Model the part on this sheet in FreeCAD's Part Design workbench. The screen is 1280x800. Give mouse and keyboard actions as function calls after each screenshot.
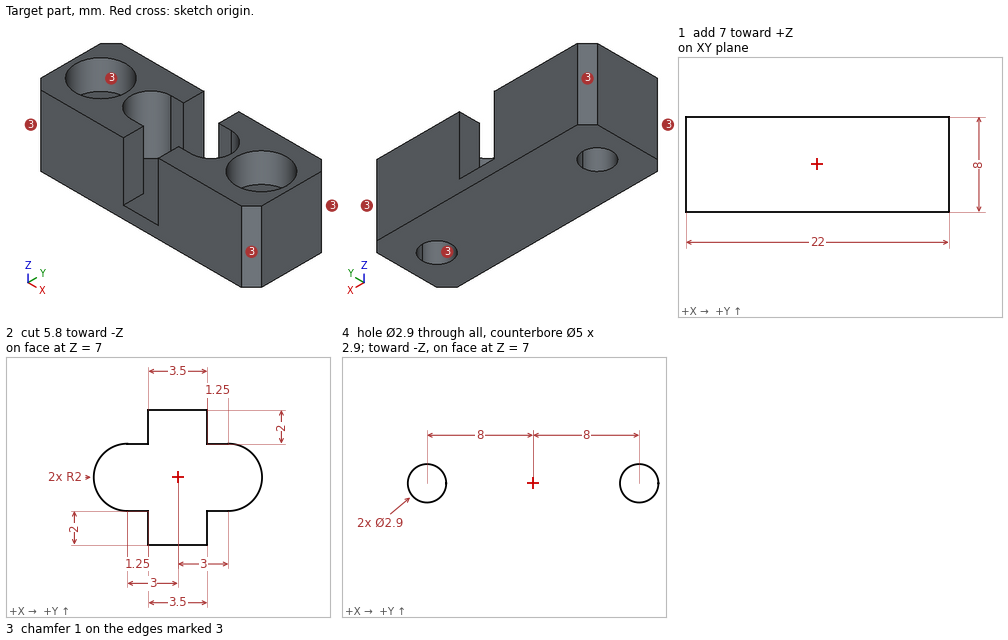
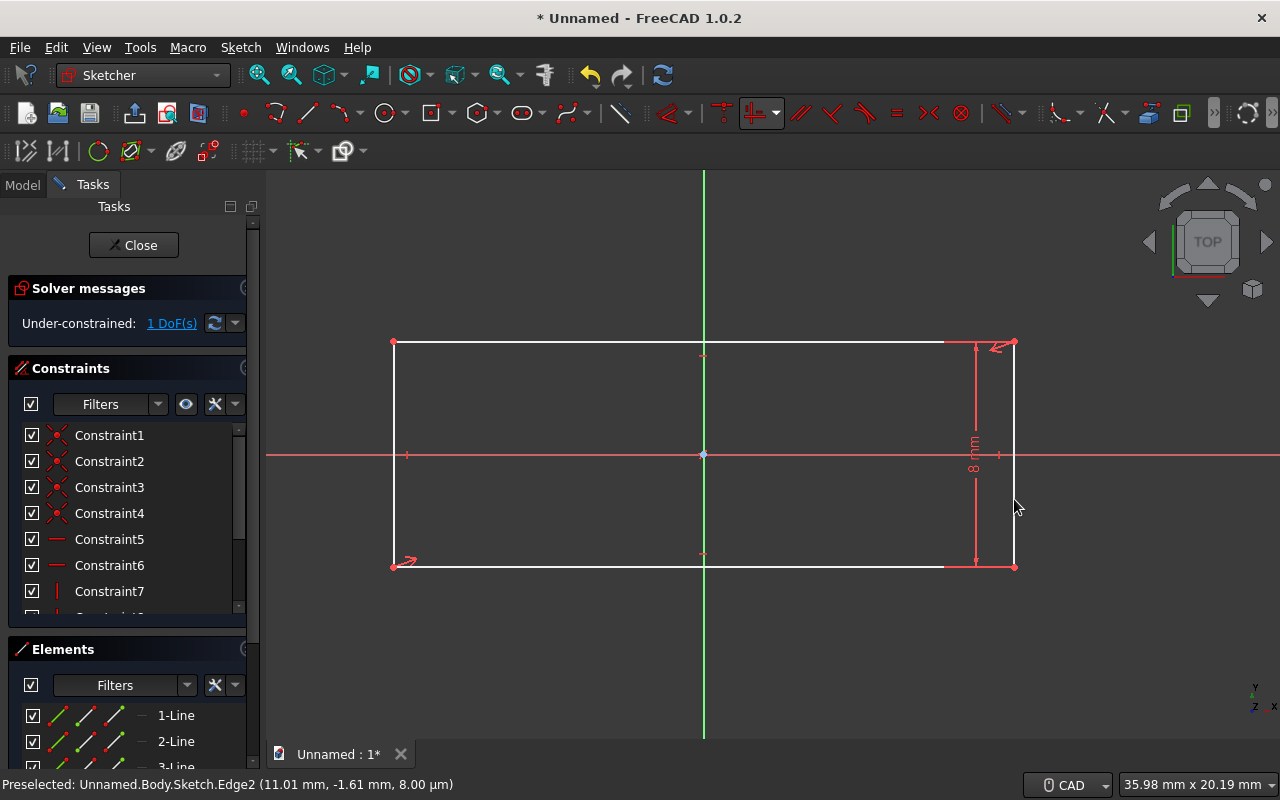
click(580, 567)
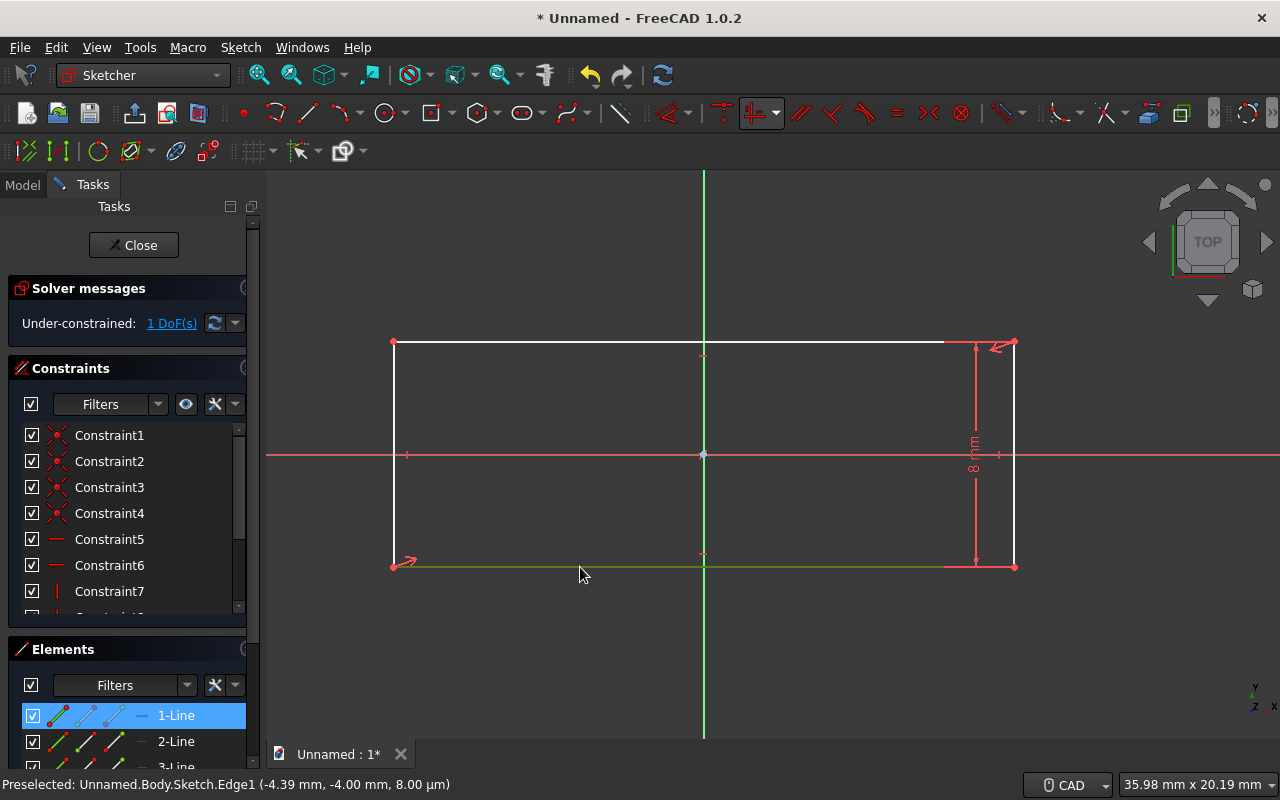
click(690, 114)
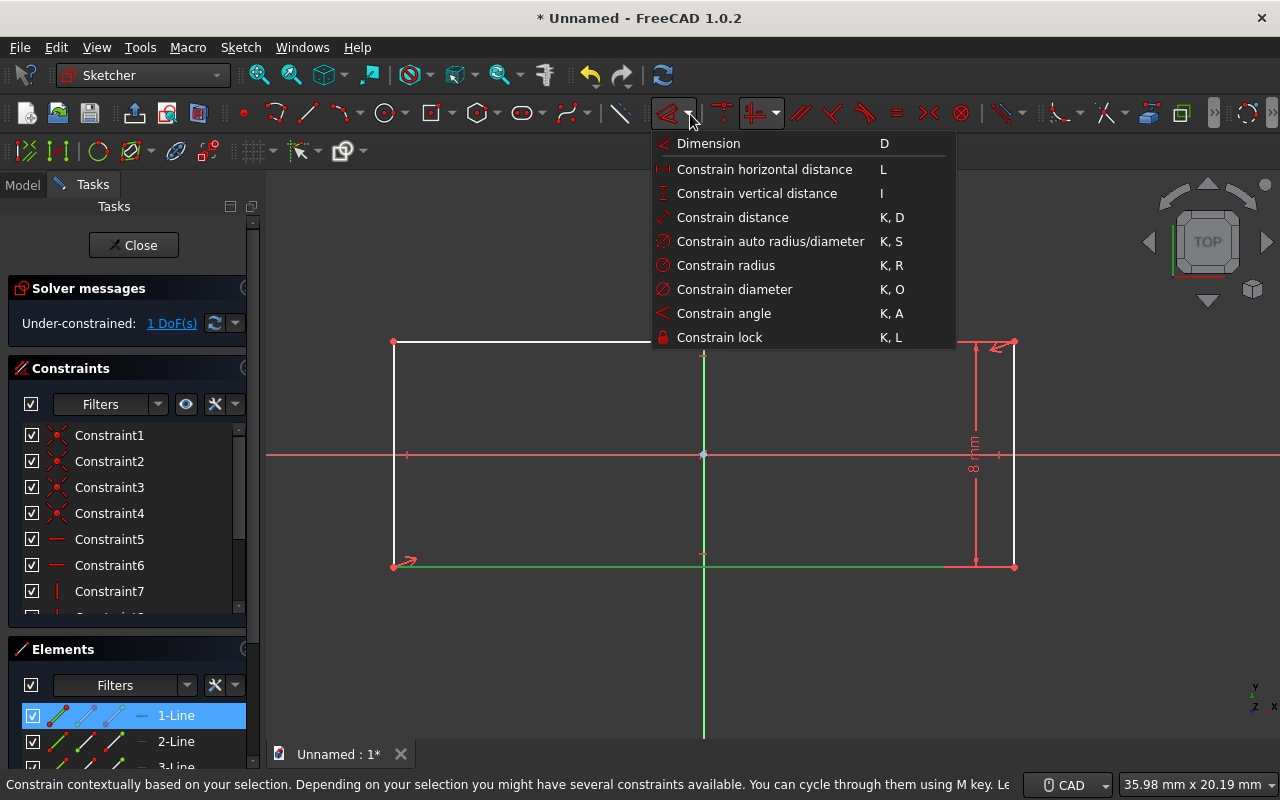
click(804, 169)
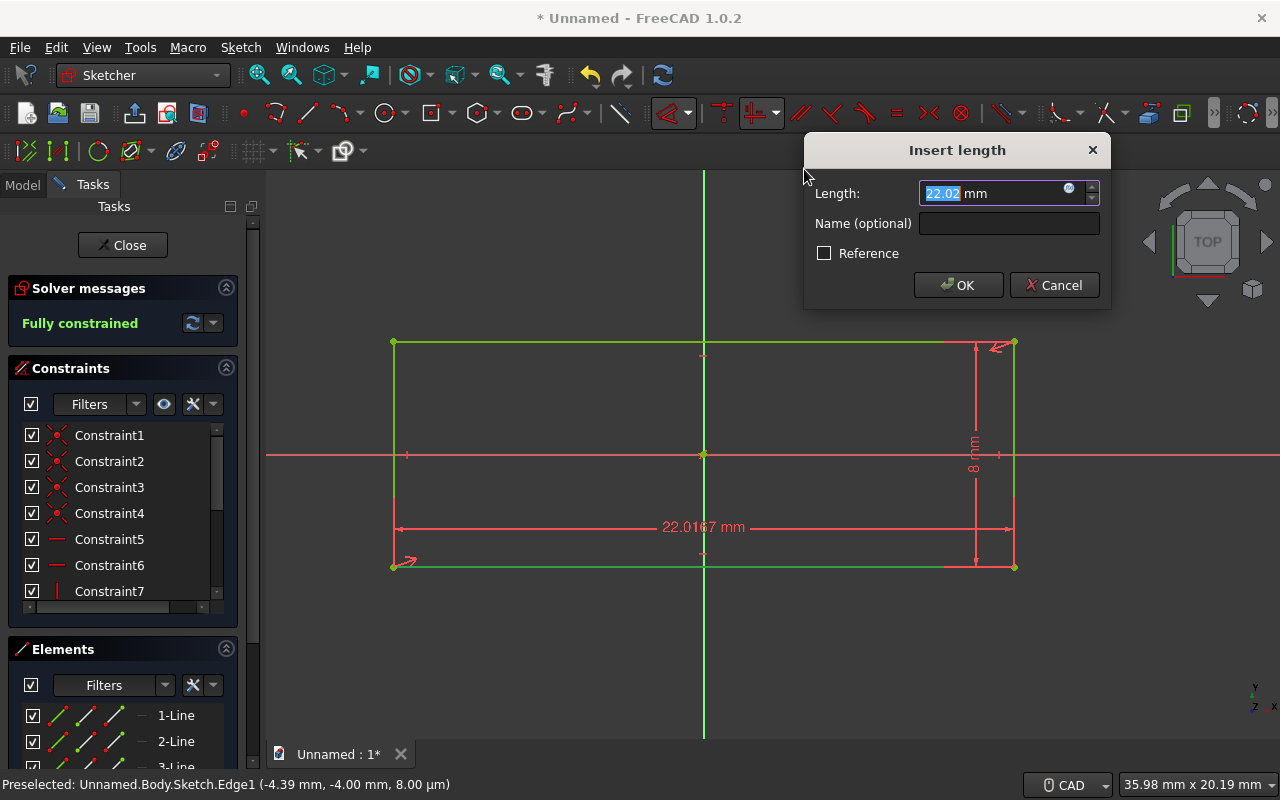
text(22)
key(Return)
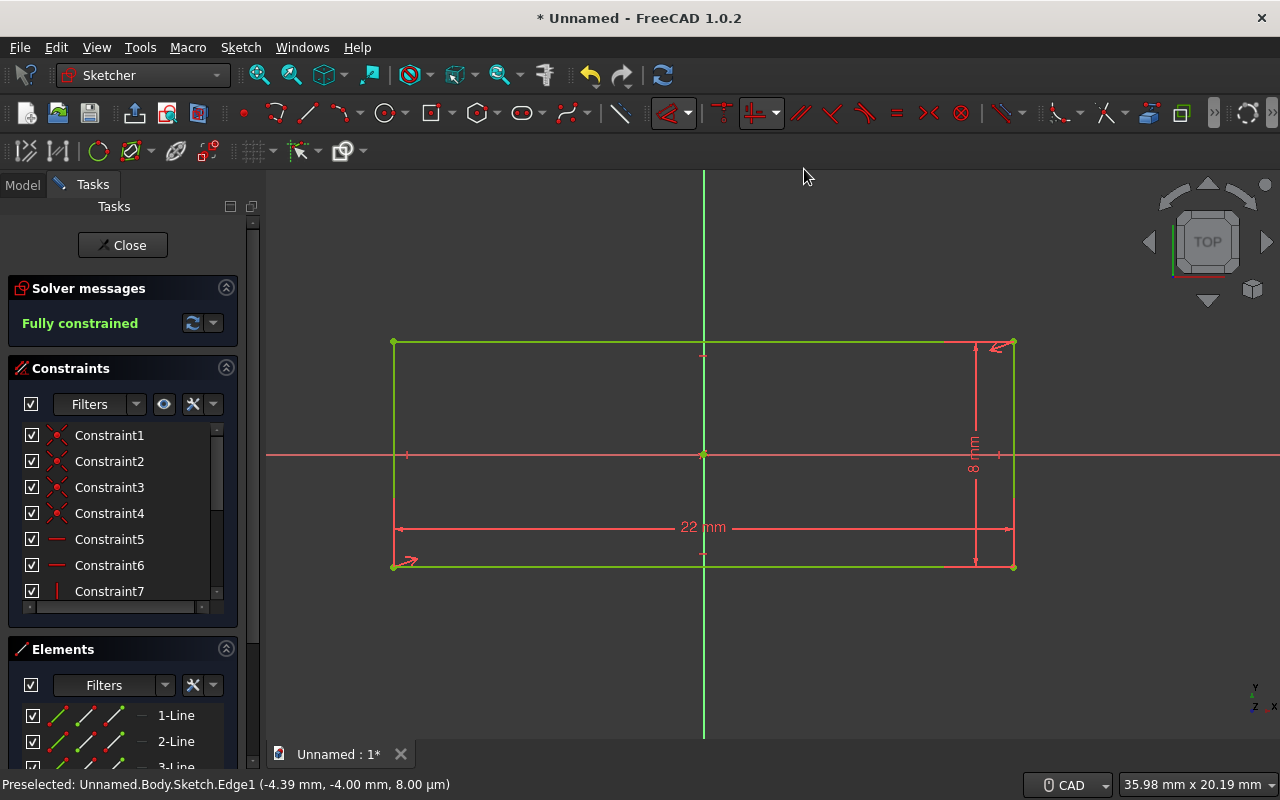
click(123, 245)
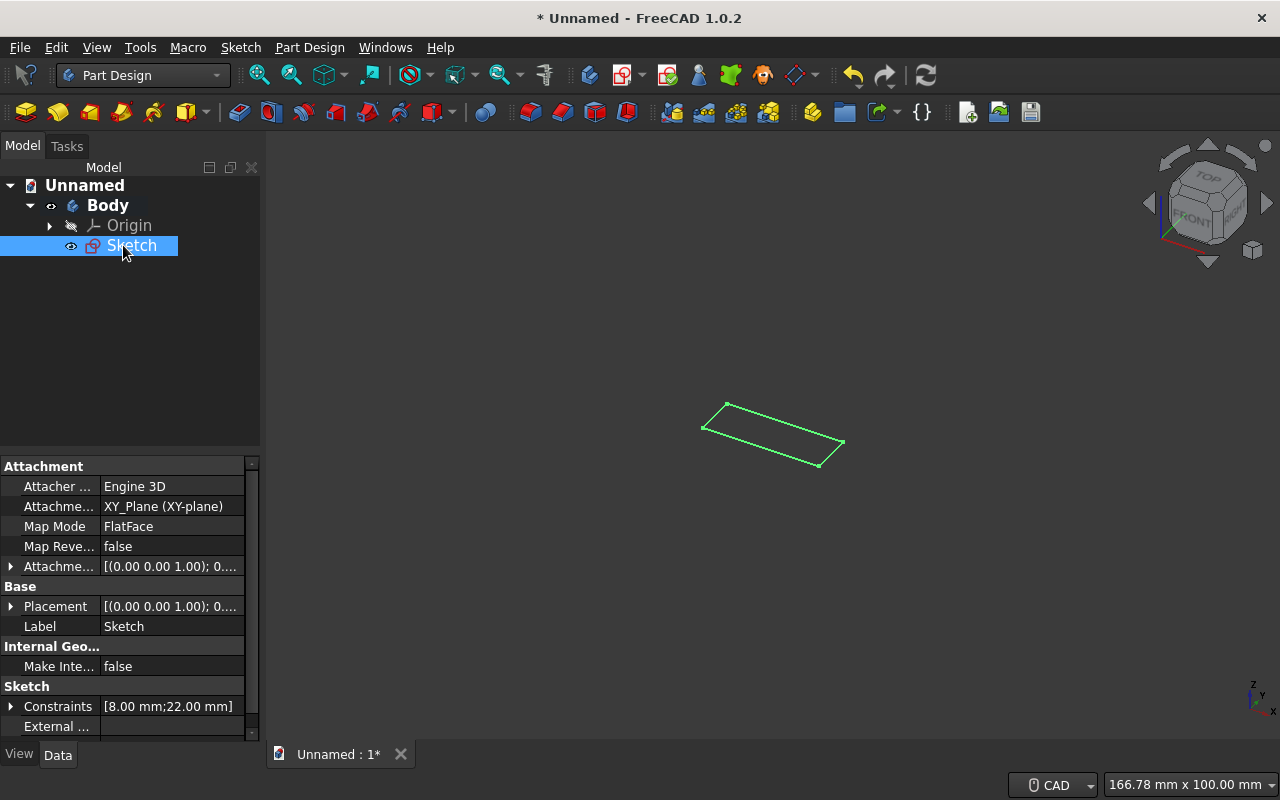
click(26, 112)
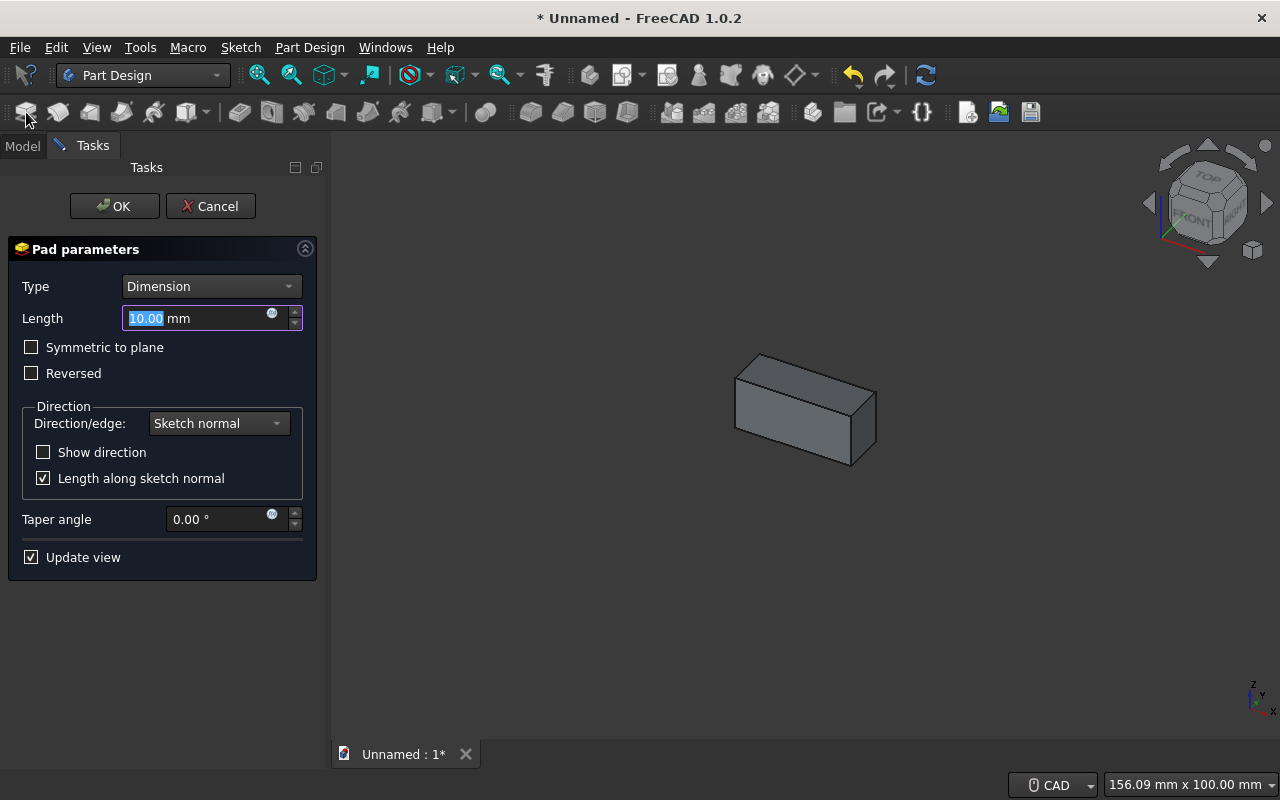
text(7)
key(Tab)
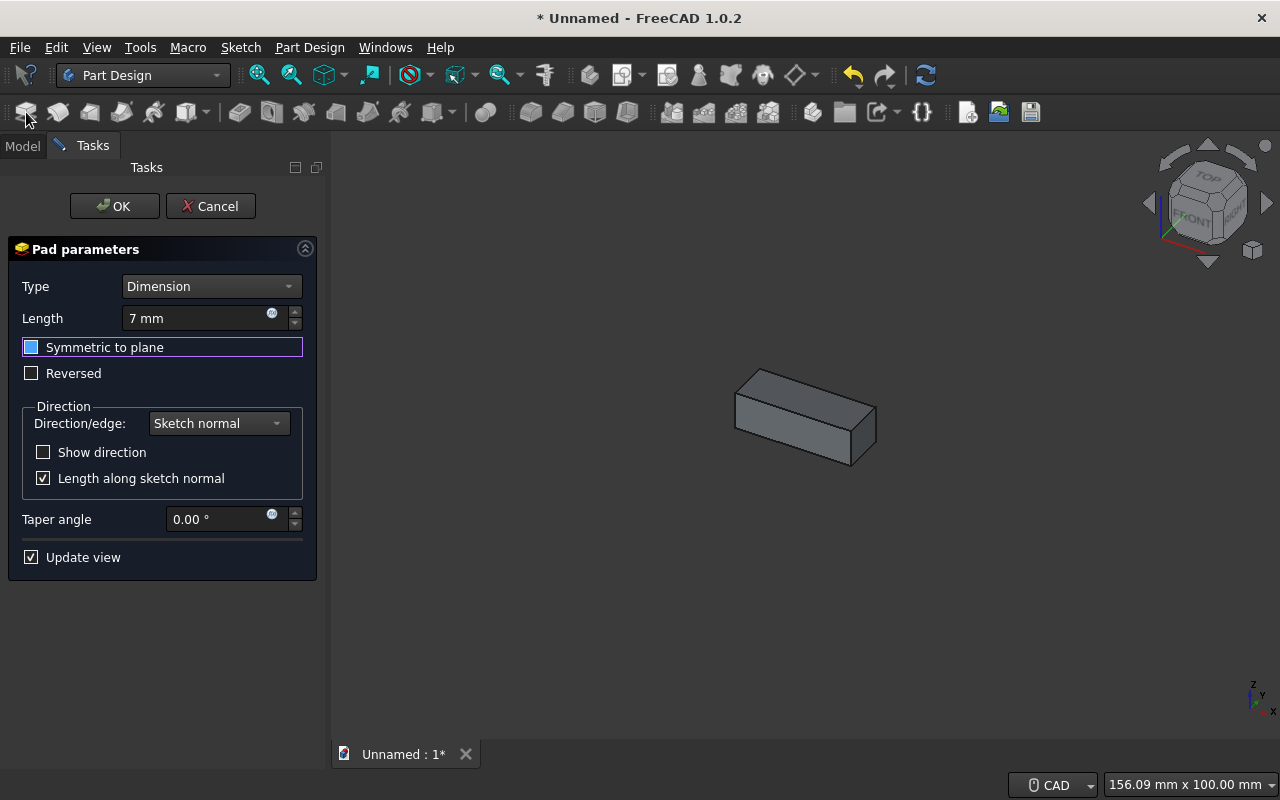
click(115, 206)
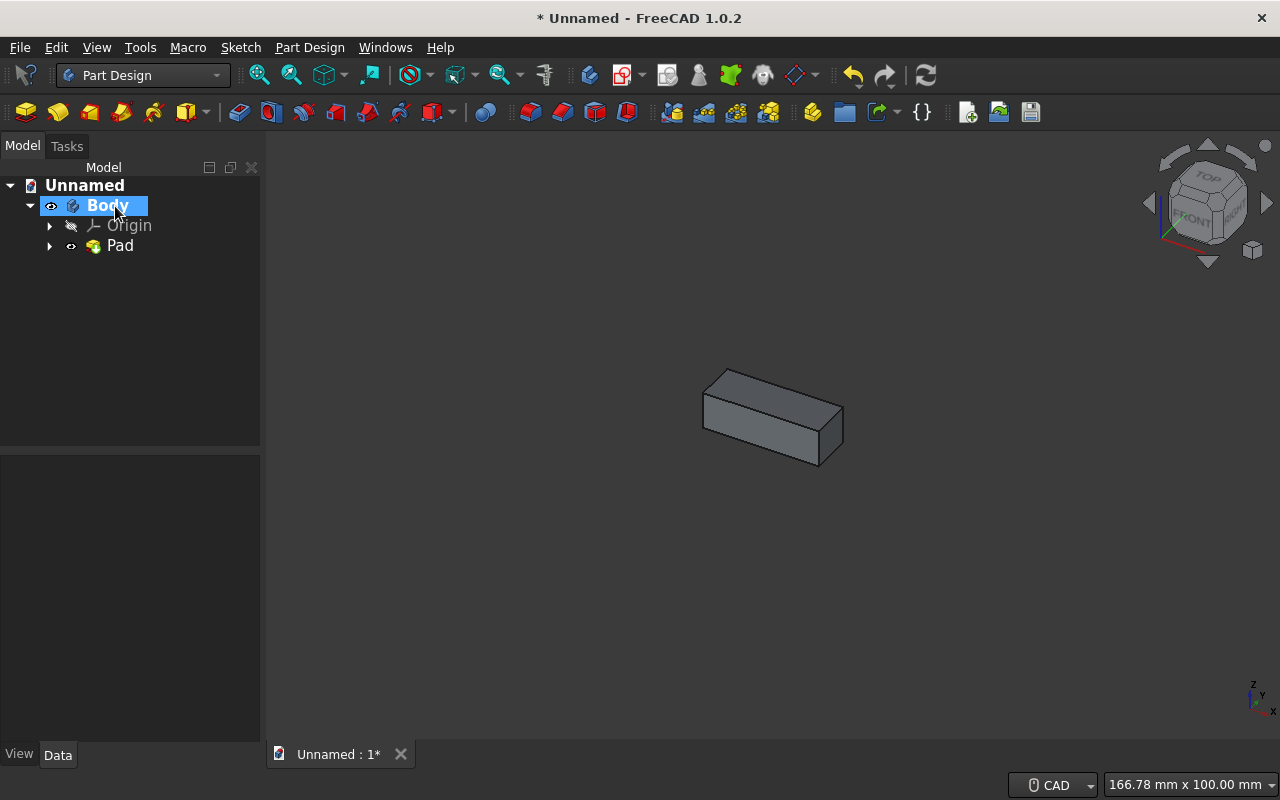
click(260, 76)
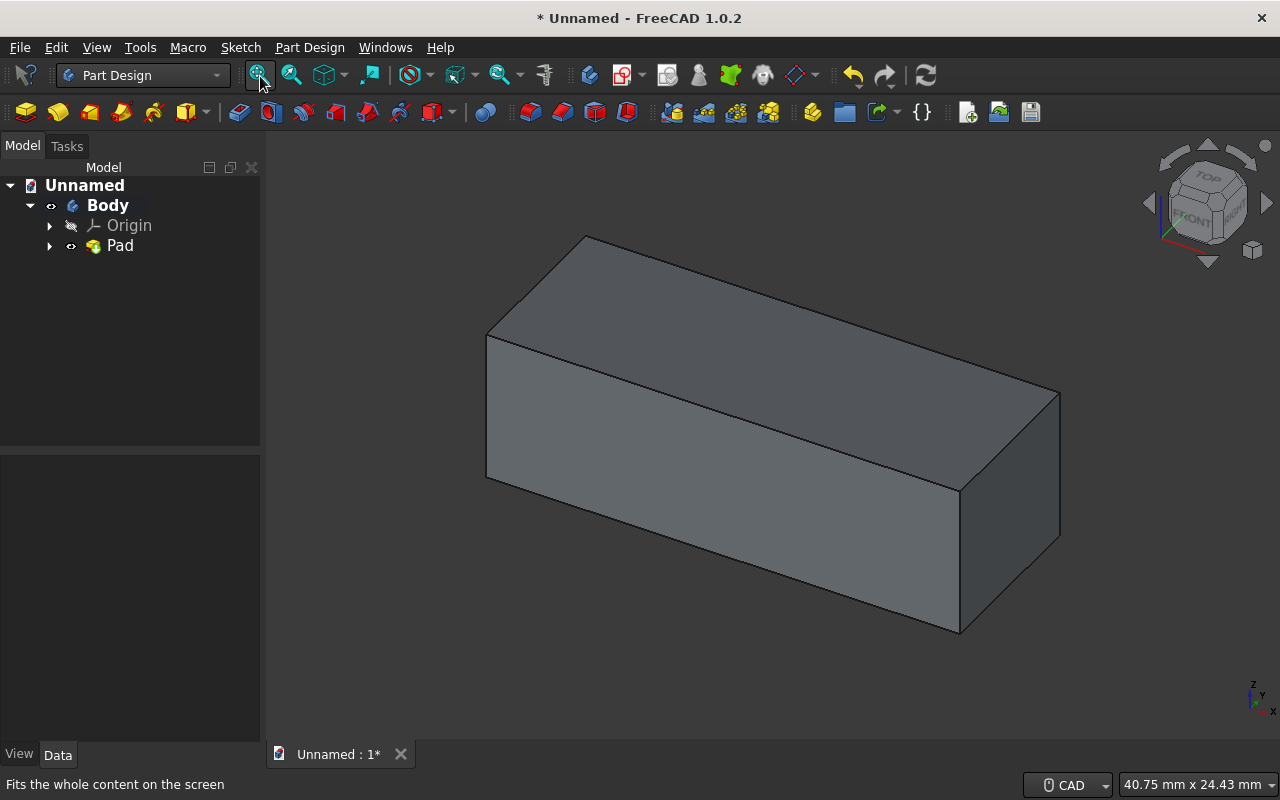
click(908, 408)